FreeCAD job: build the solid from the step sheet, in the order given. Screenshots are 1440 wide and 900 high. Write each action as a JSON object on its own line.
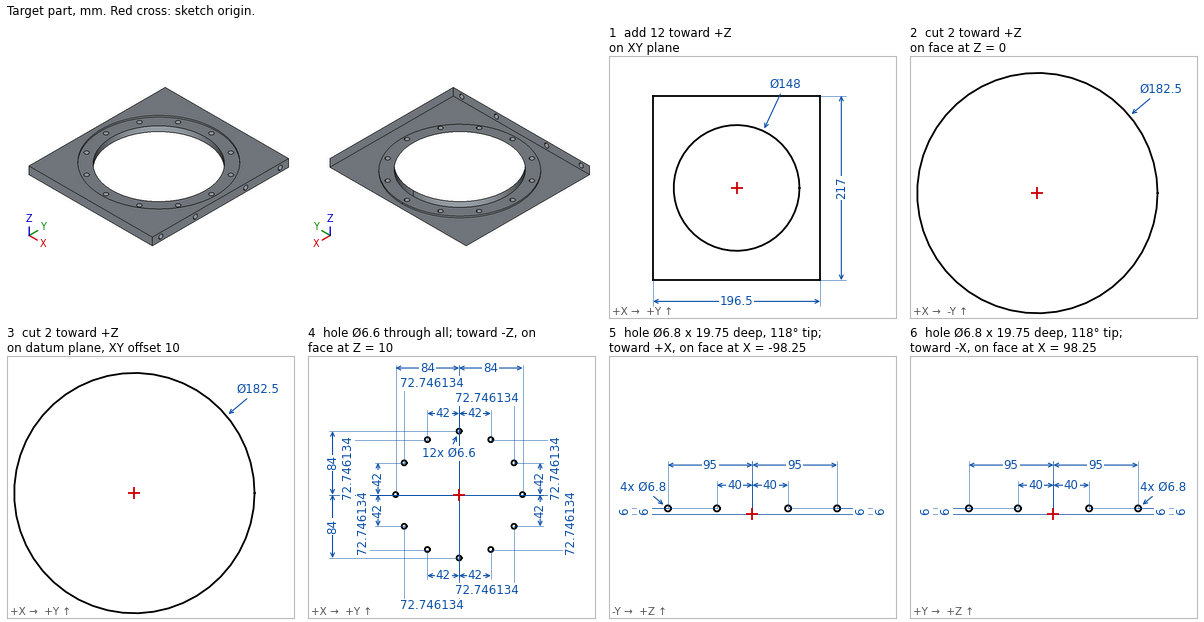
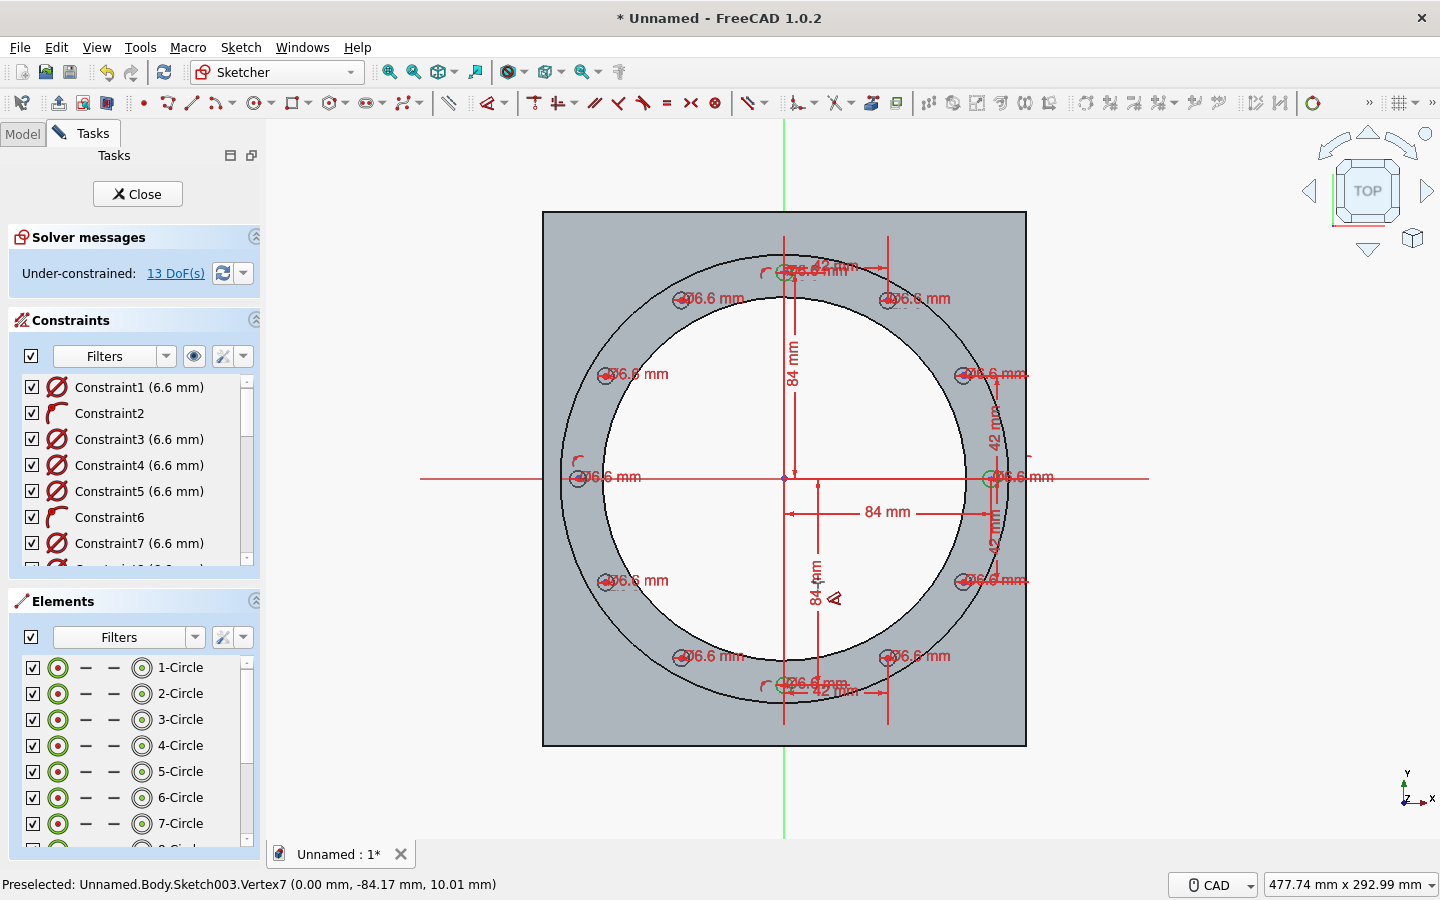
{"action": "left_click", "coordinate": [681, 658]}
{"action": "left_click", "coordinate": [733, 692]}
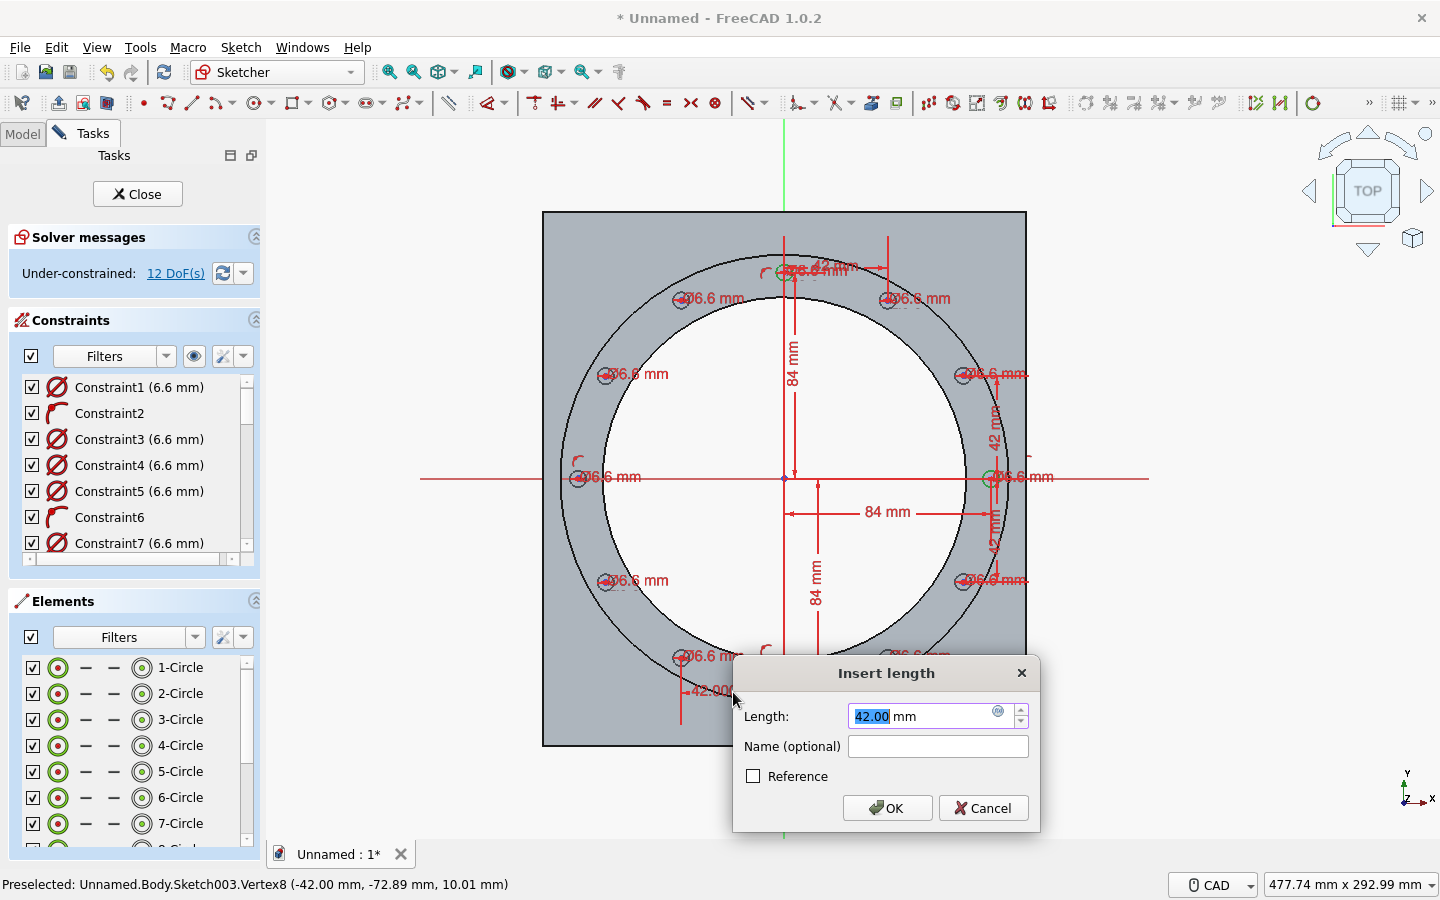
{"action": "type", "text": "42"}
{"action": "key", "text": "Return"}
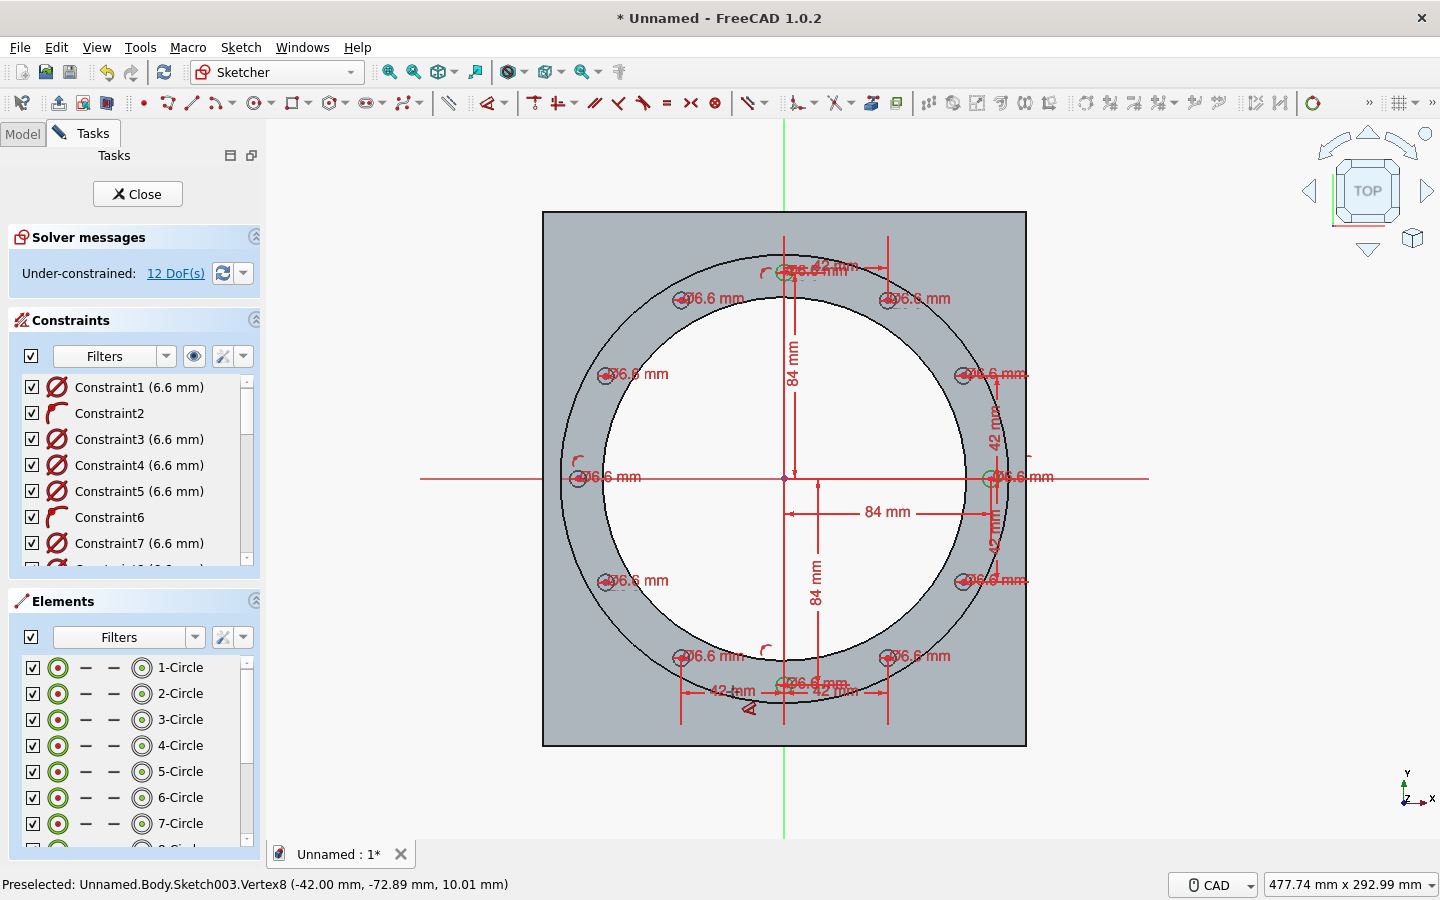
{"action": "left_click", "coordinate": [606, 583]}
{"action": "left_click", "coordinate": [572, 531]}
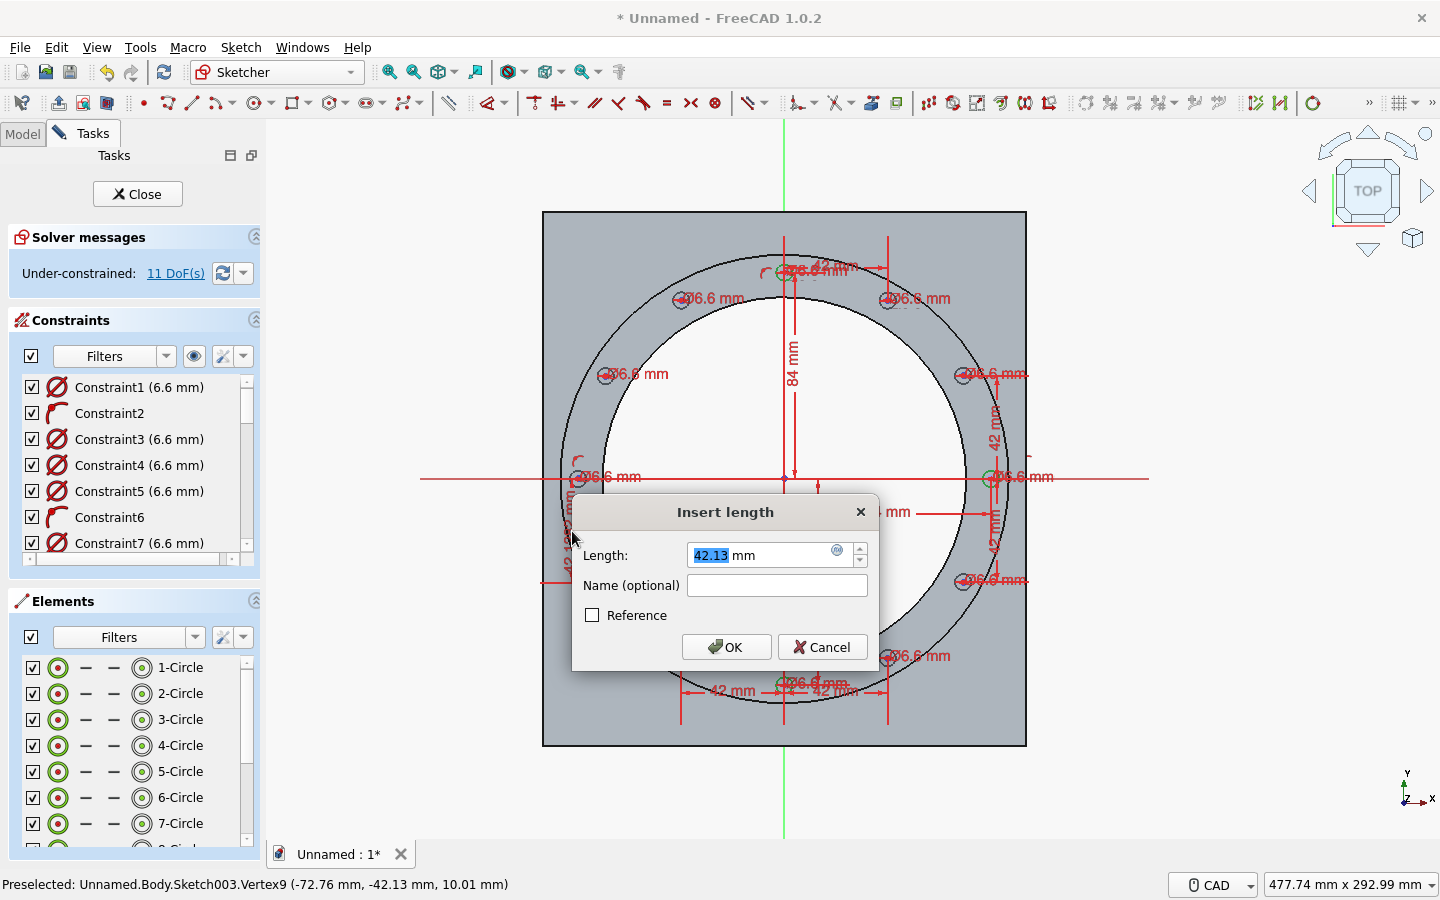
{"action": "type", "text": "42"}
{"action": "key", "text": "Return"}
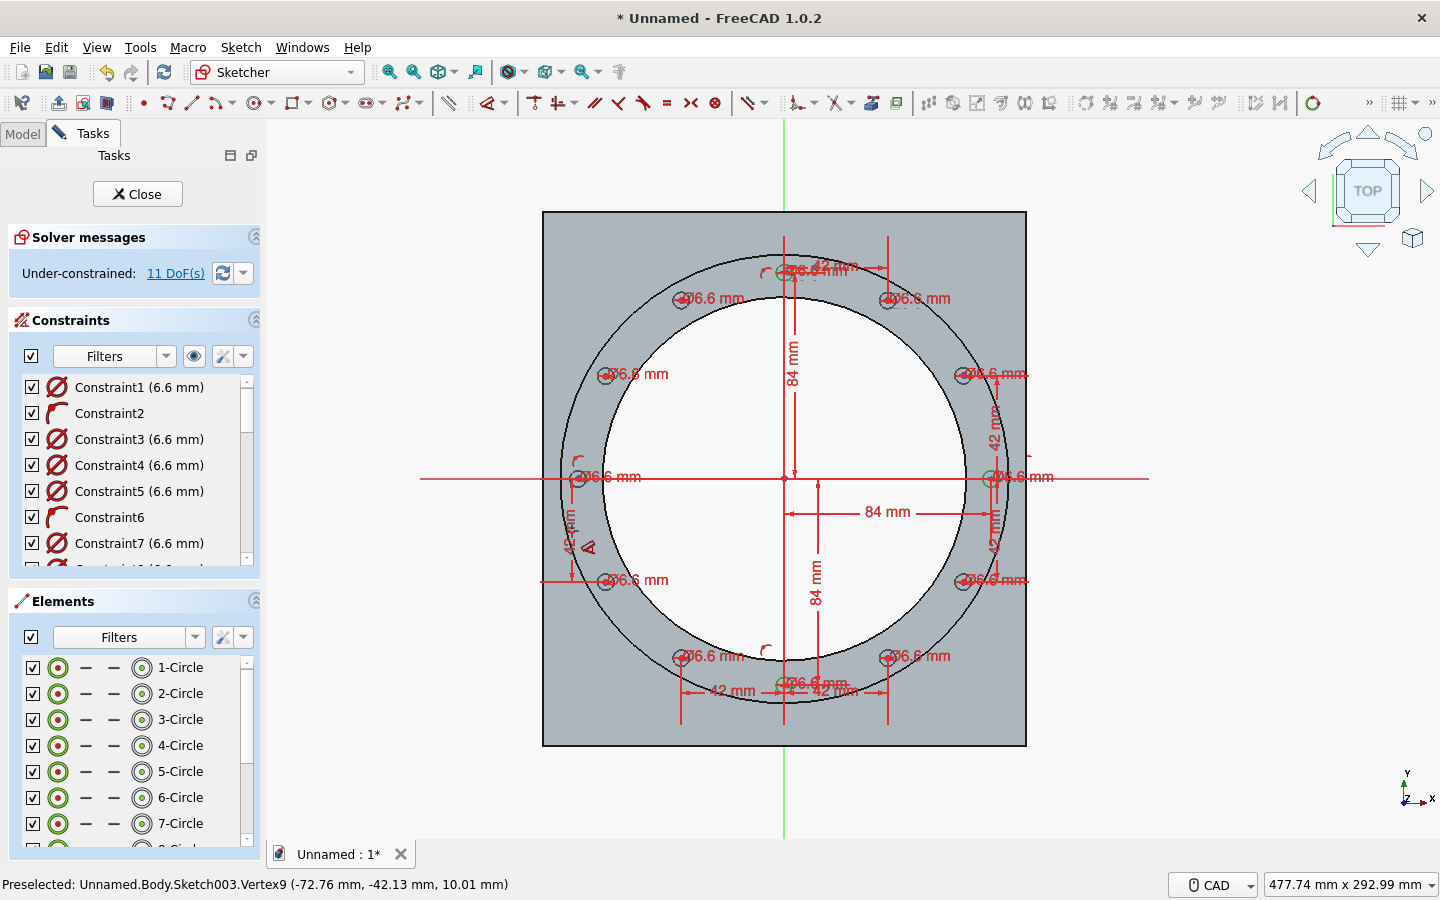
{"action": "left_click", "coordinate": [578, 479]}
{"action": "left_click", "coordinate": [681, 513]}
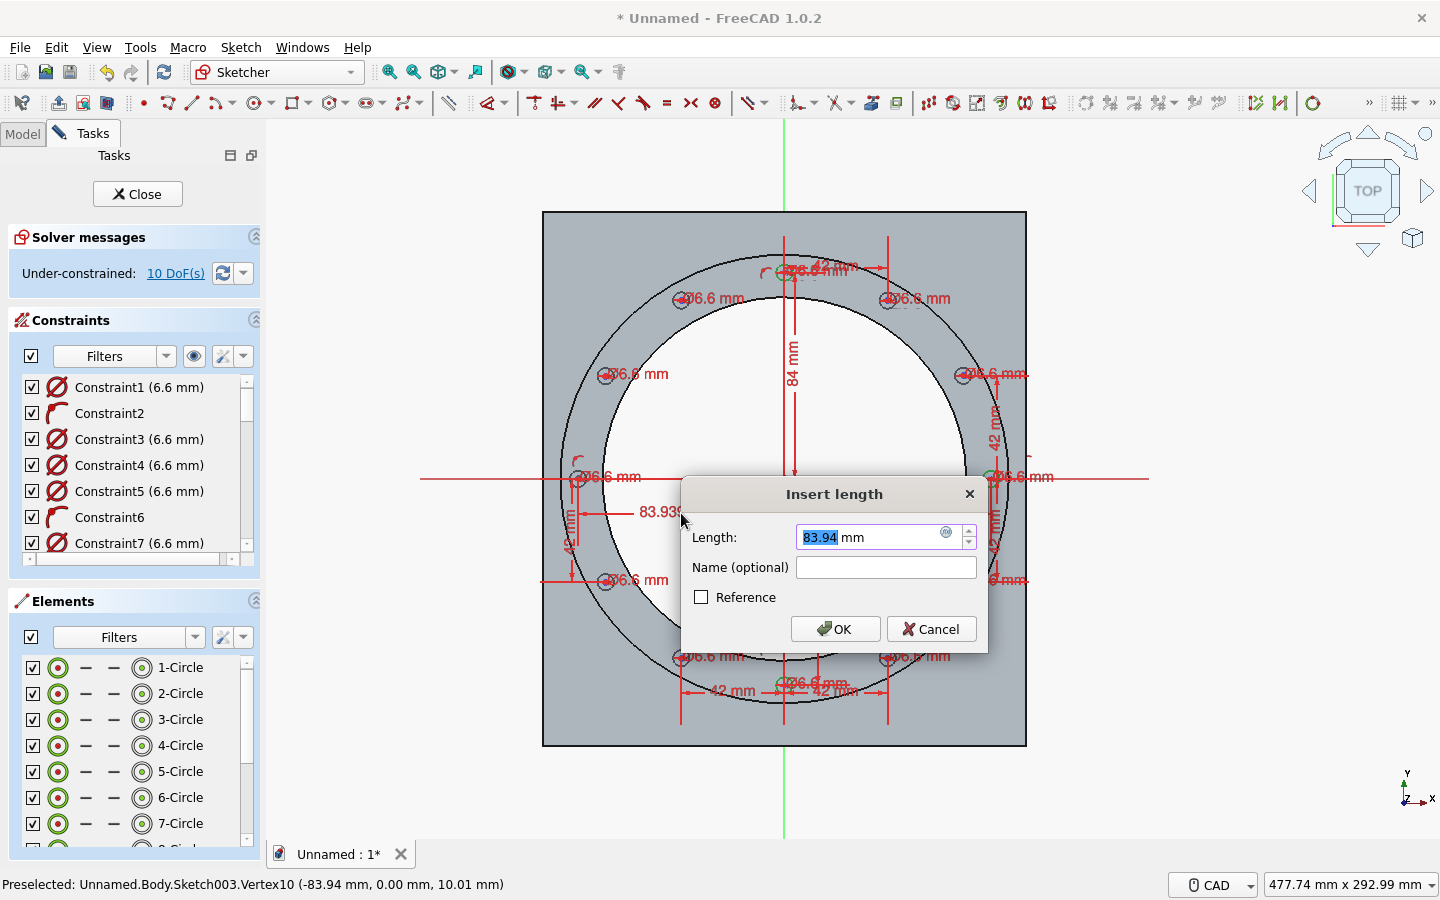
{"action": "type", "text": "84"}
{"action": "key", "text": "Return"}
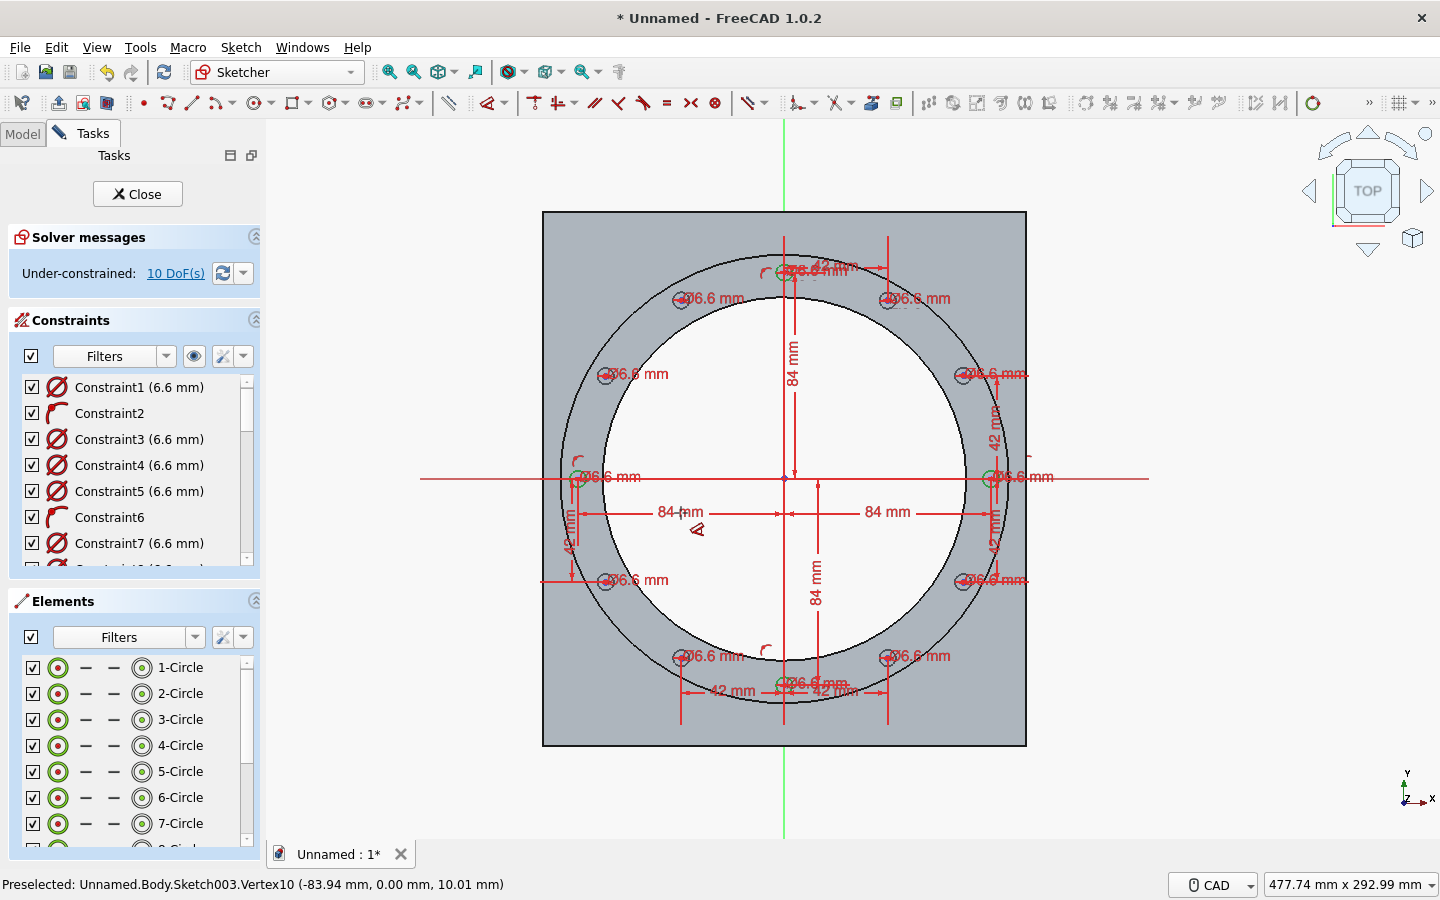
{"action": "left_click", "coordinate": [606, 376]}
{"action": "left_click", "coordinate": [572, 428]}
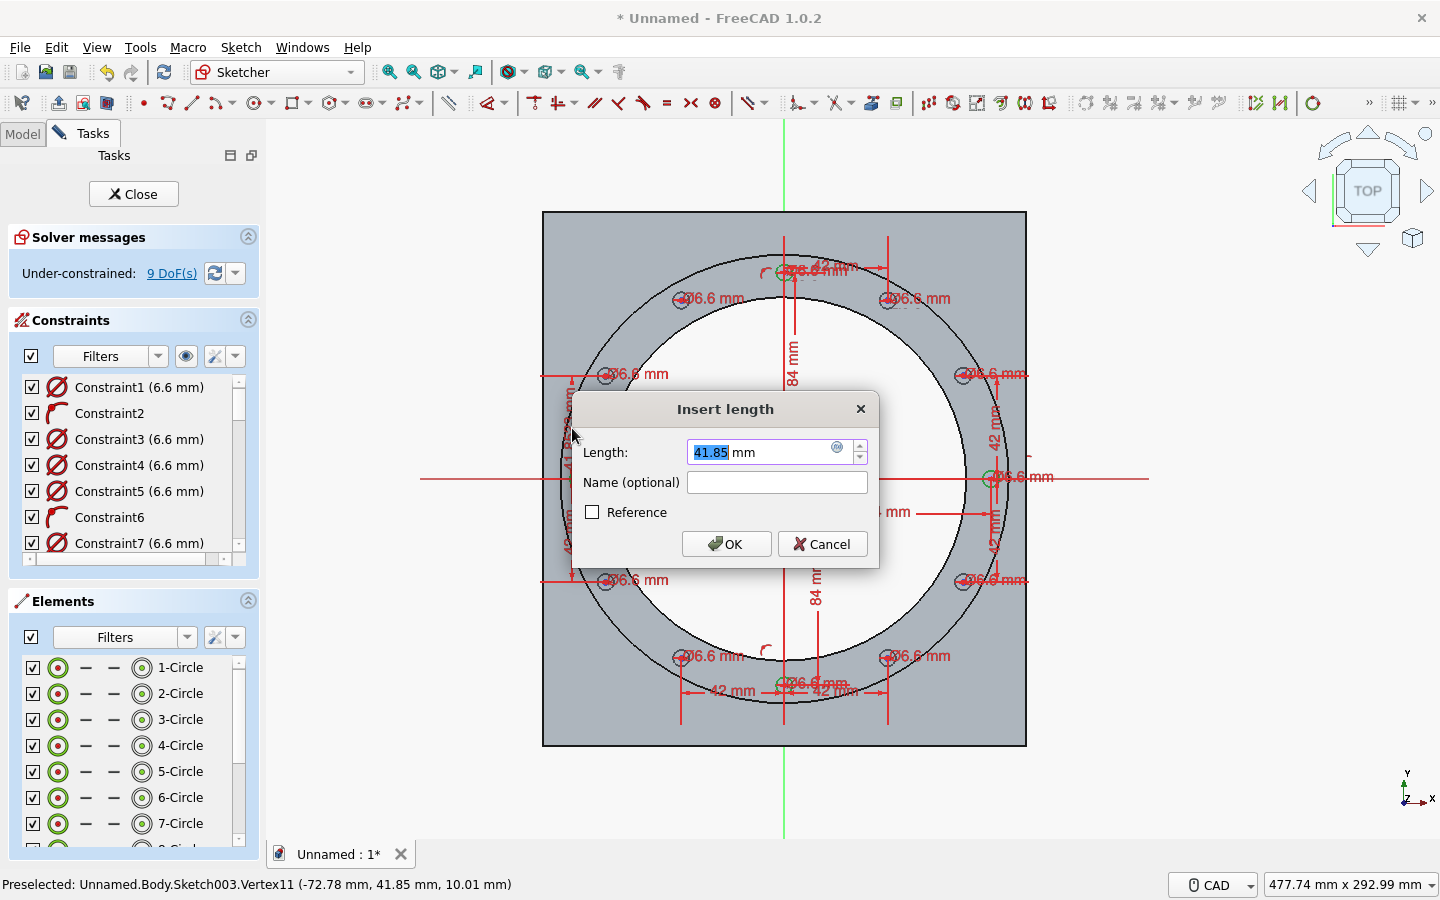
{"action": "type", "text": "42"}
{"action": "key", "text": "Return"}